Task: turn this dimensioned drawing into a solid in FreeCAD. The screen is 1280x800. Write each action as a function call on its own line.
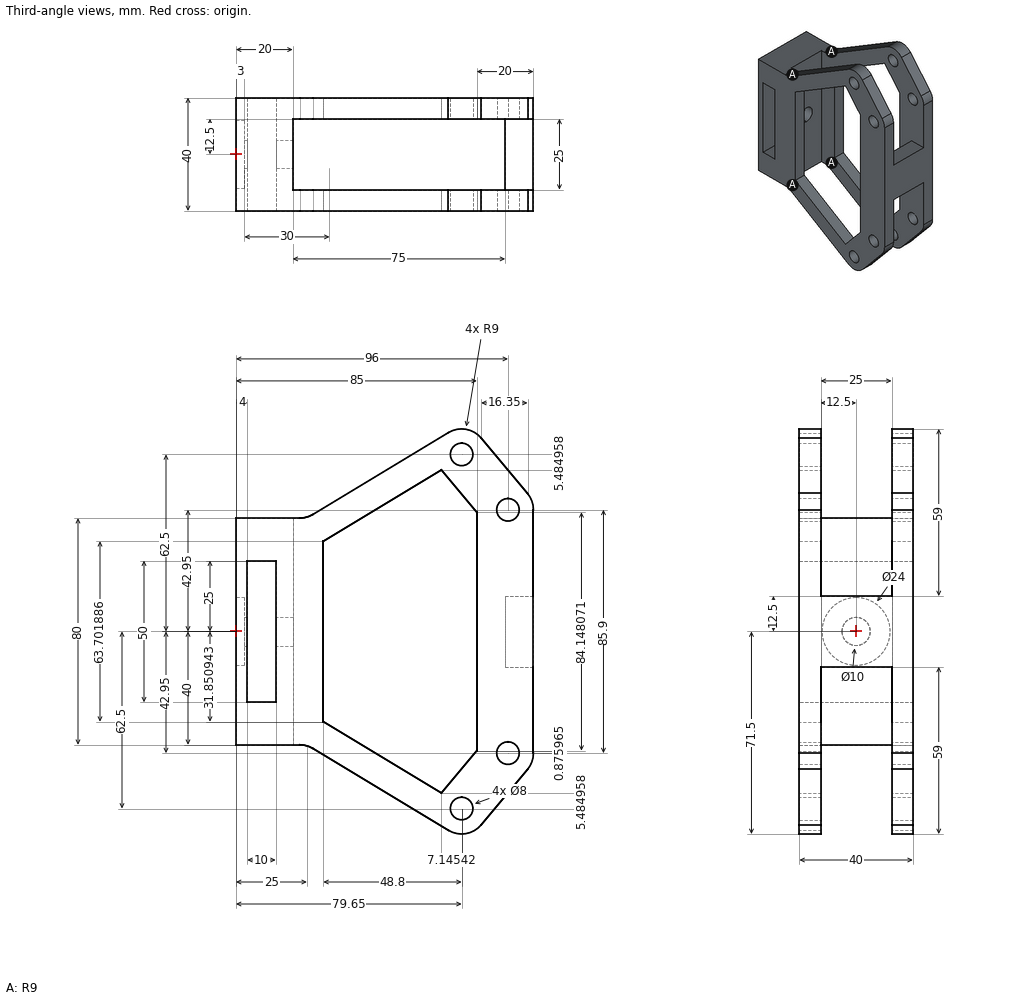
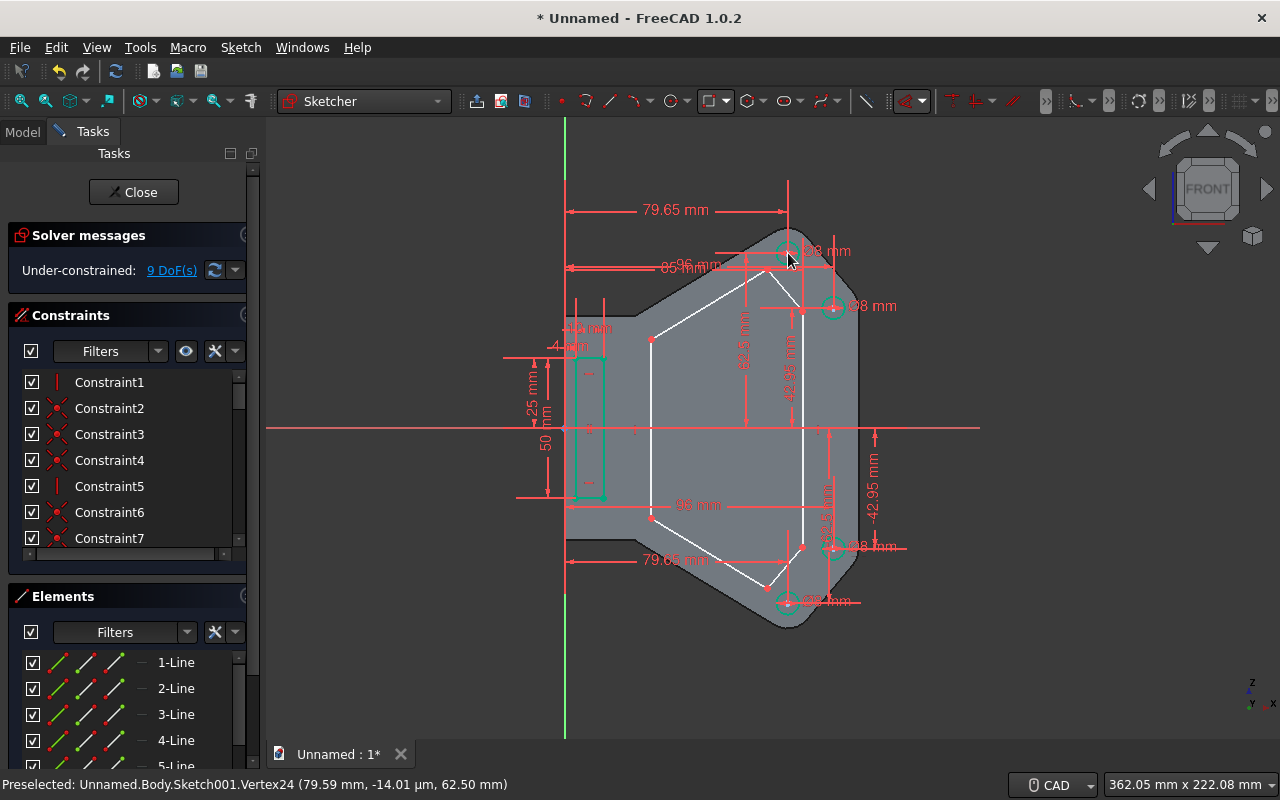
click(651, 518)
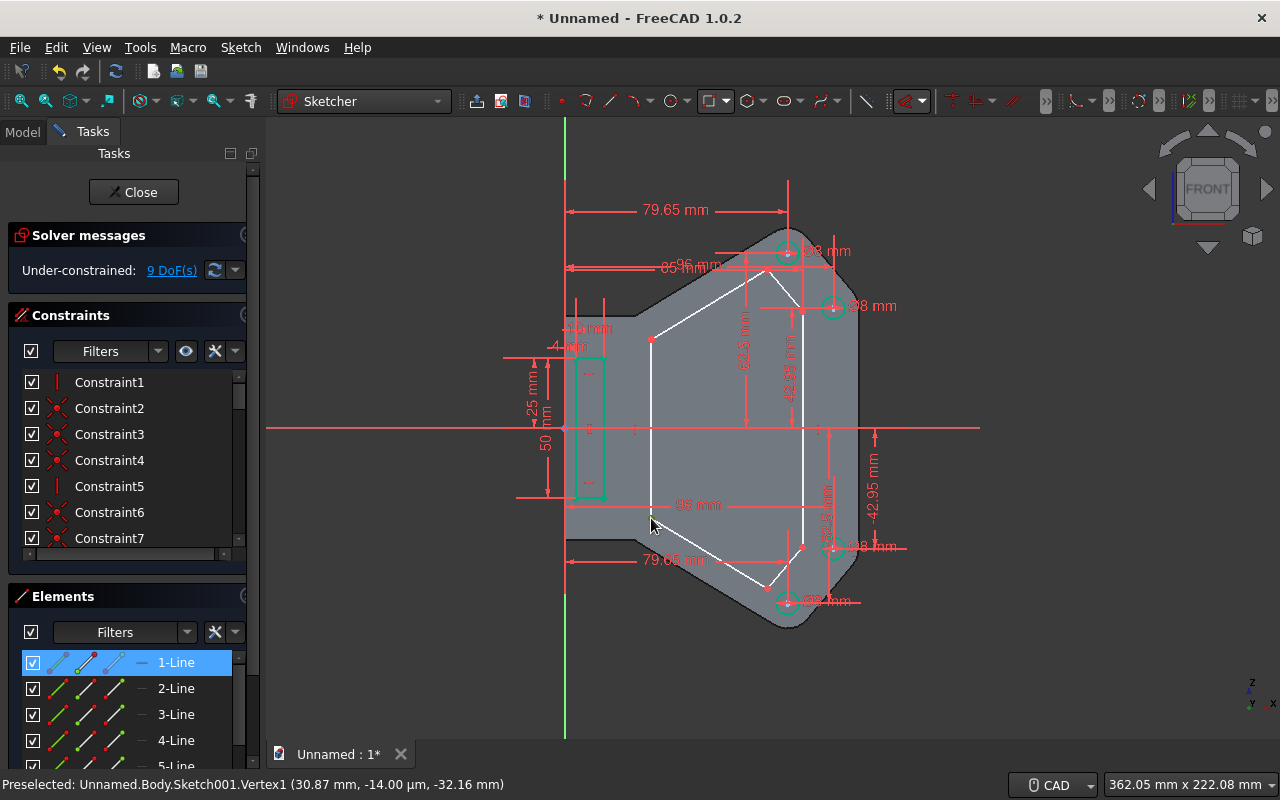
click(788, 603)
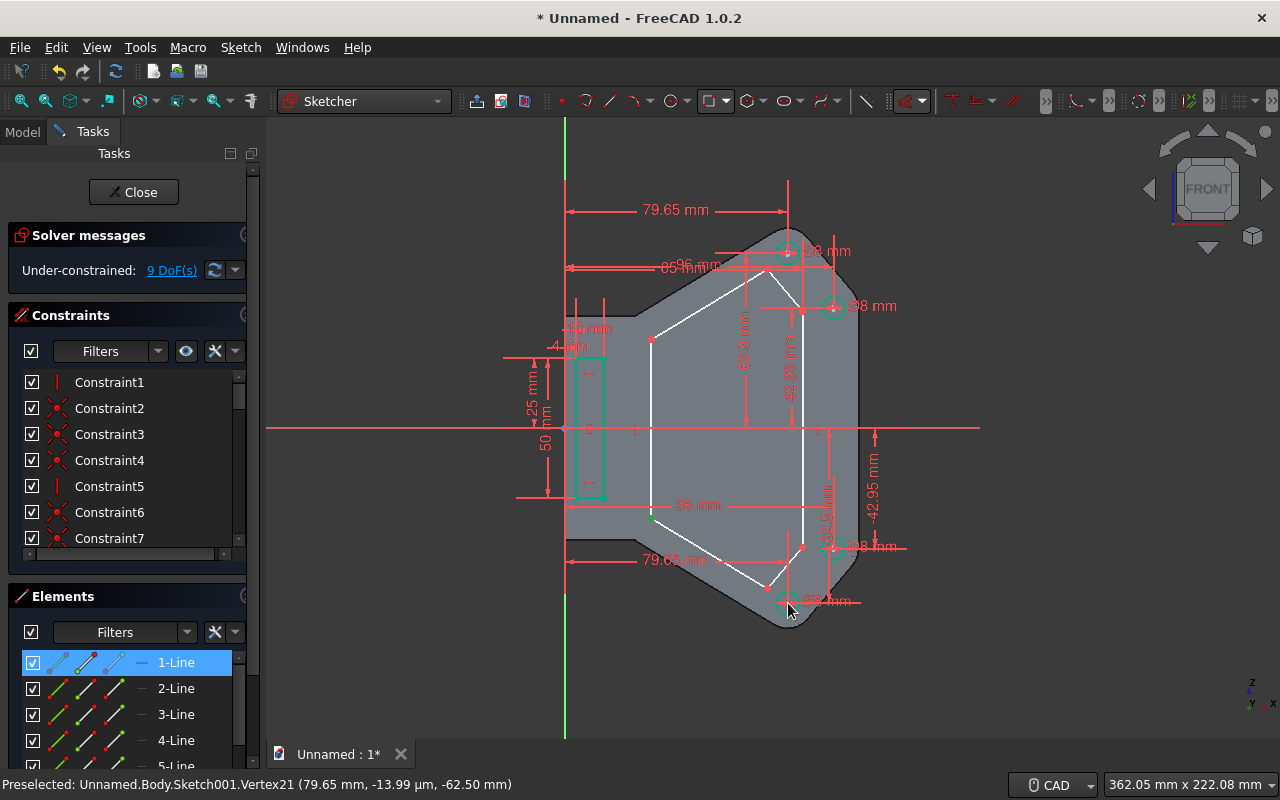
click(924, 102)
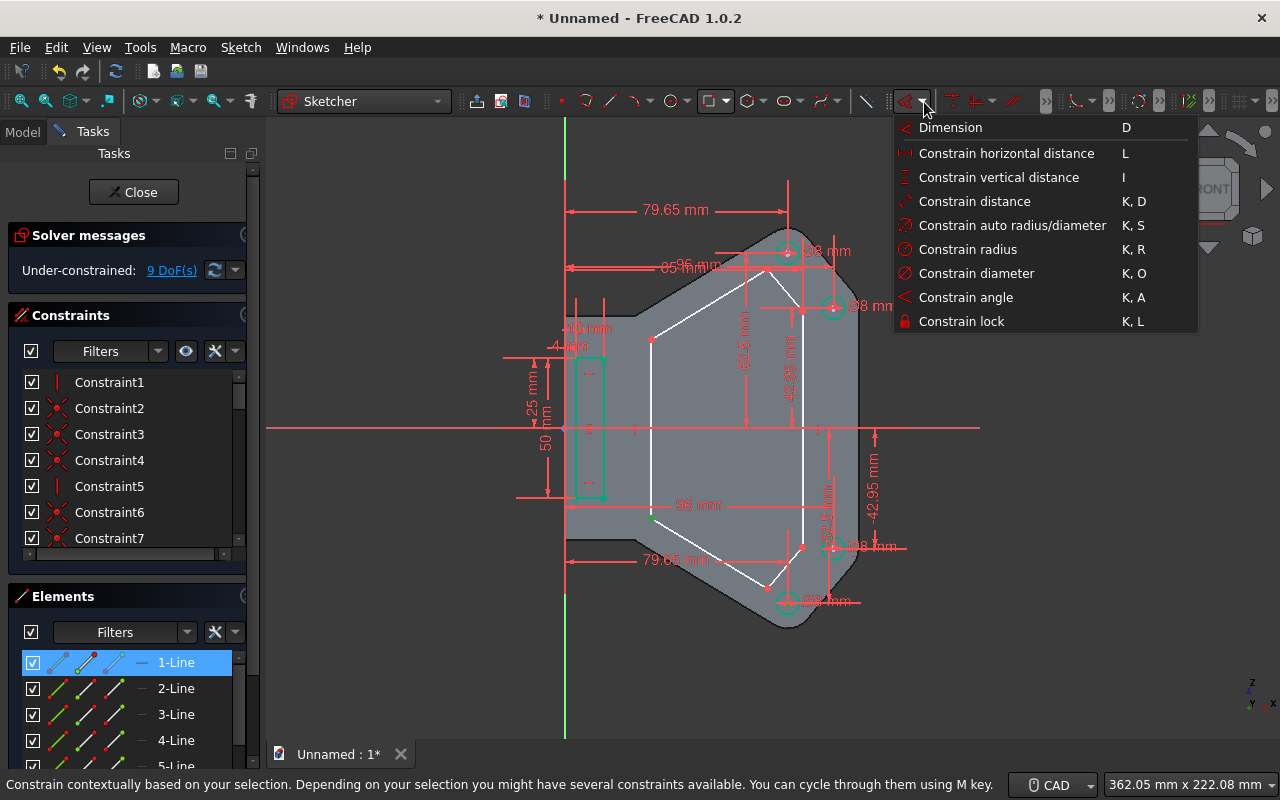
click(1046, 153)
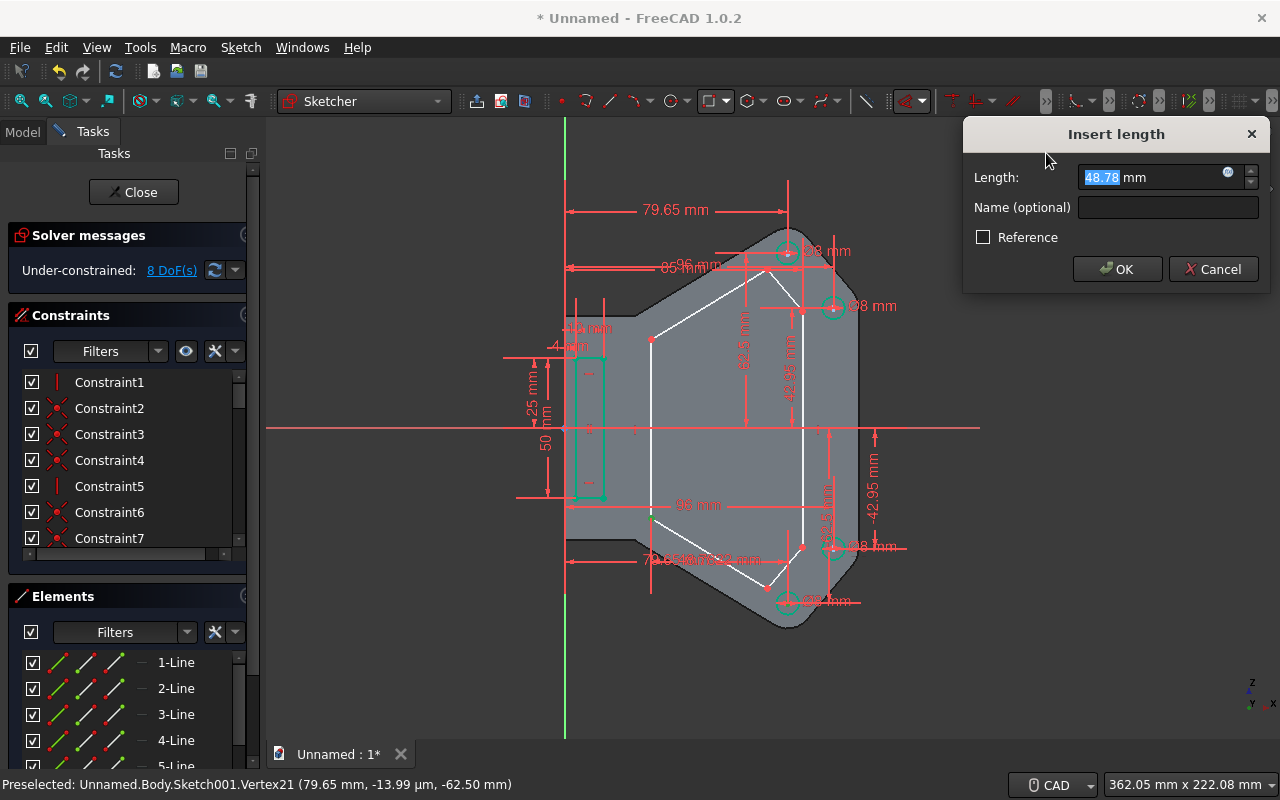
text(48.8)
key(Return)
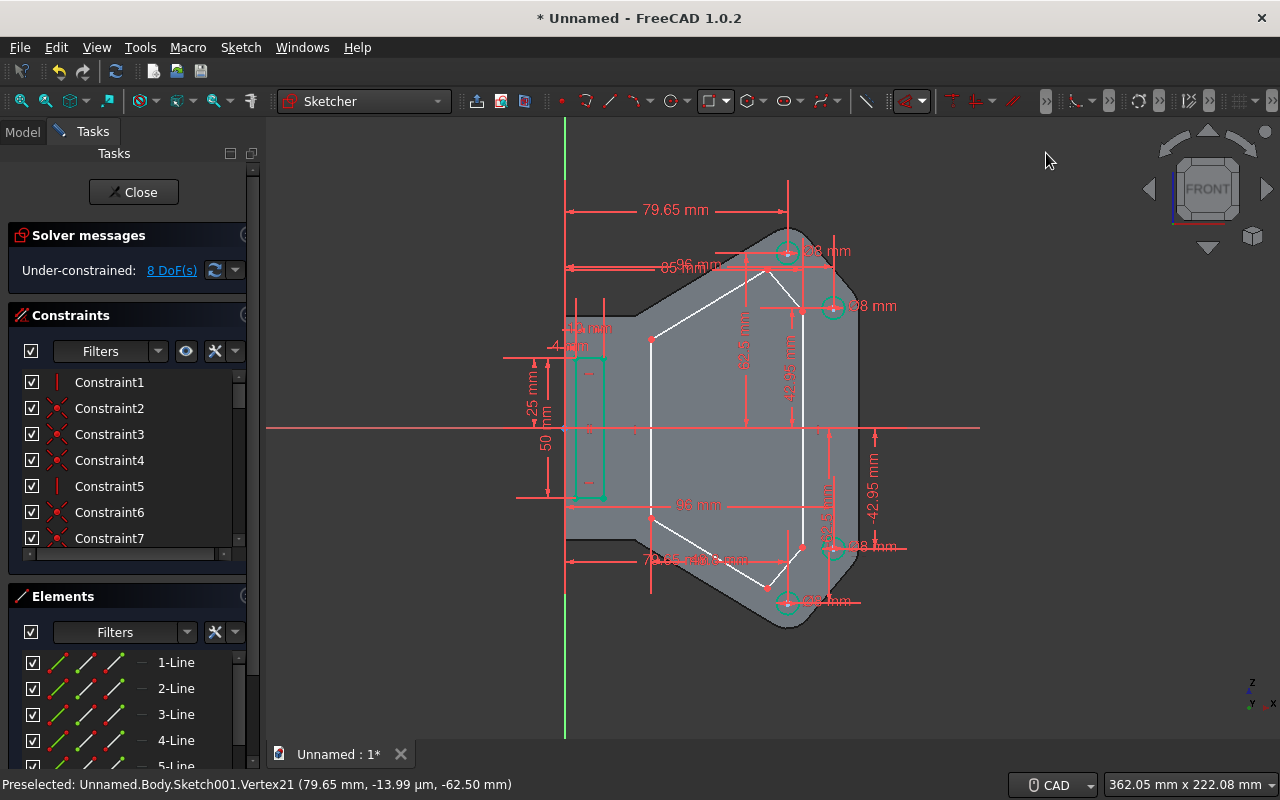
scroll(767, 589, up, 4)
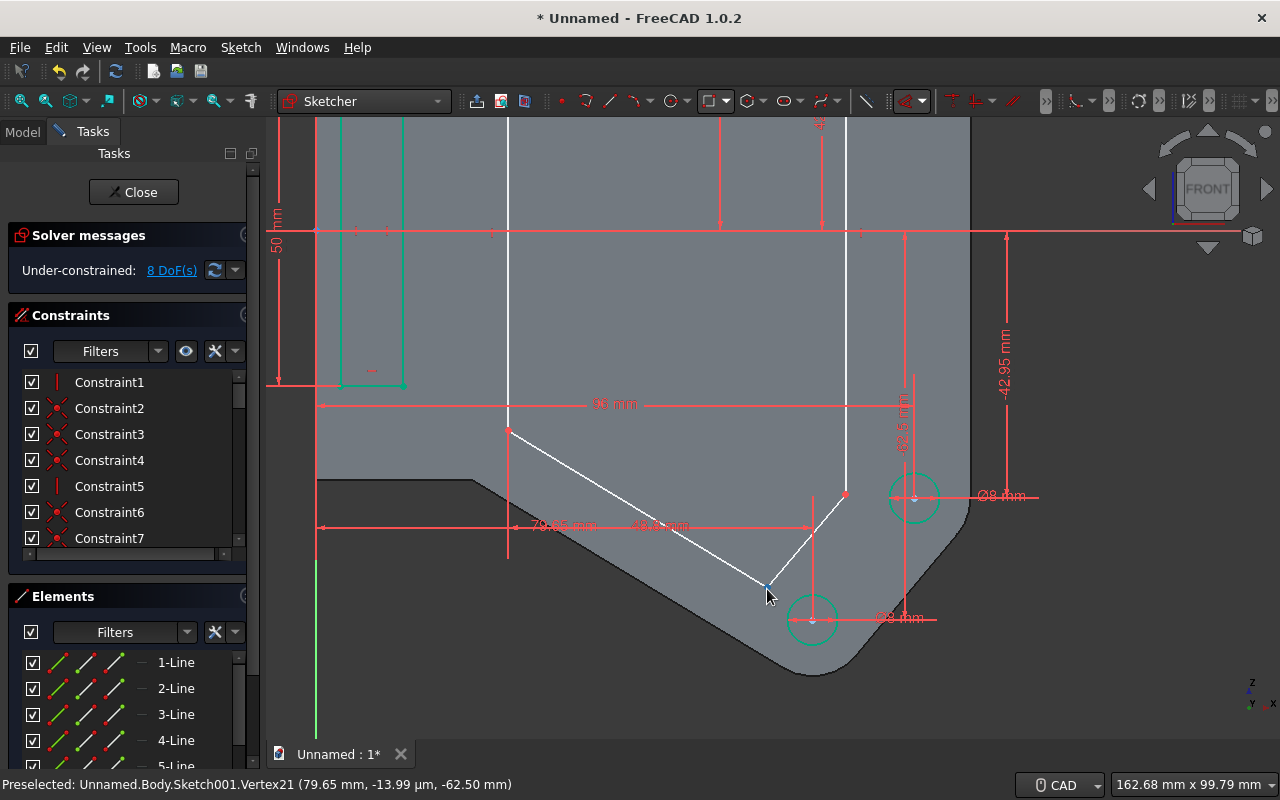
click(767, 588)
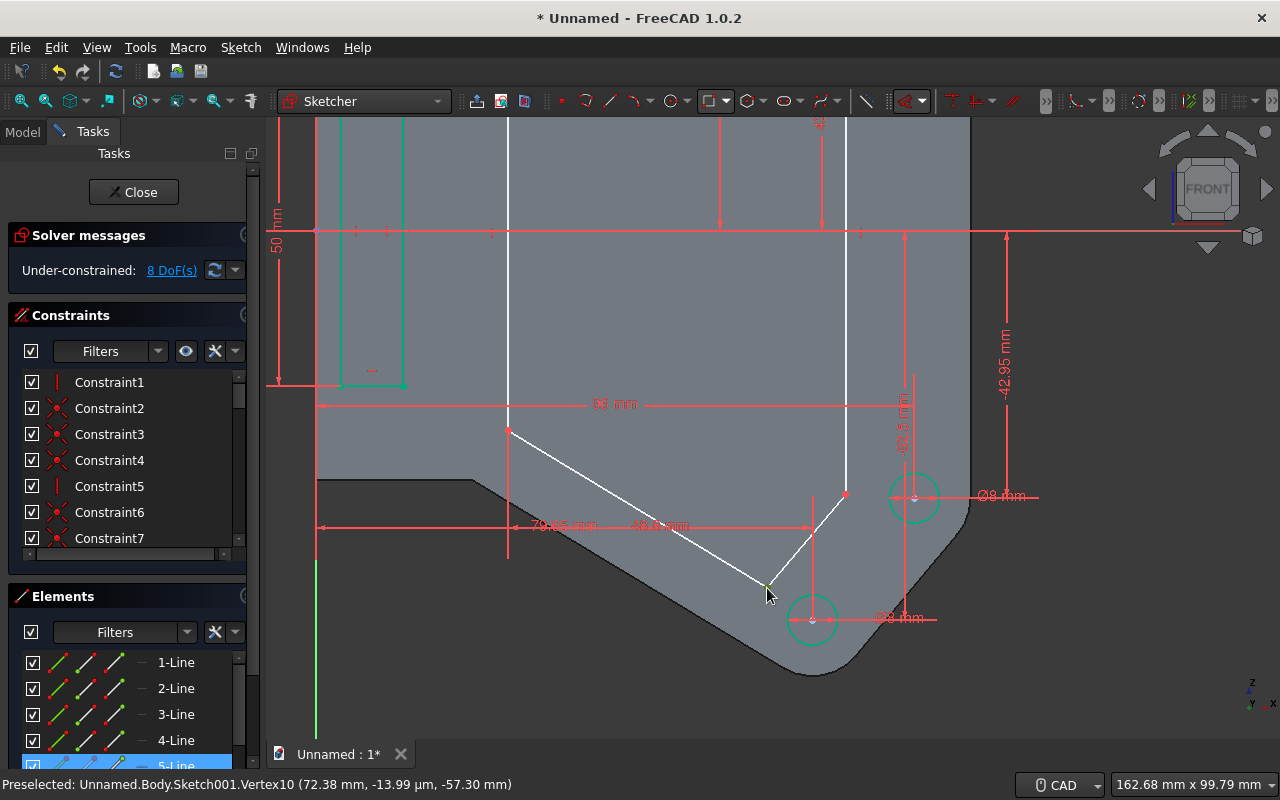
click(813, 620)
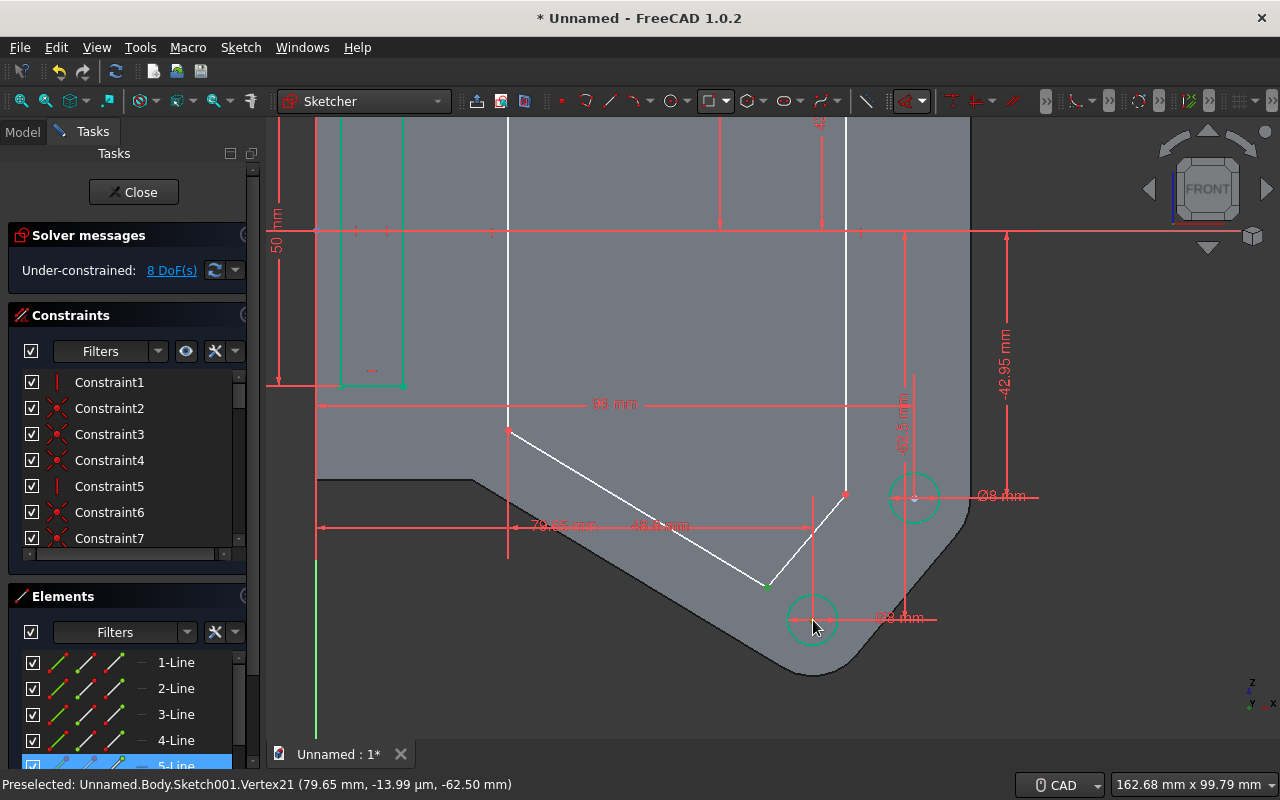
key(l)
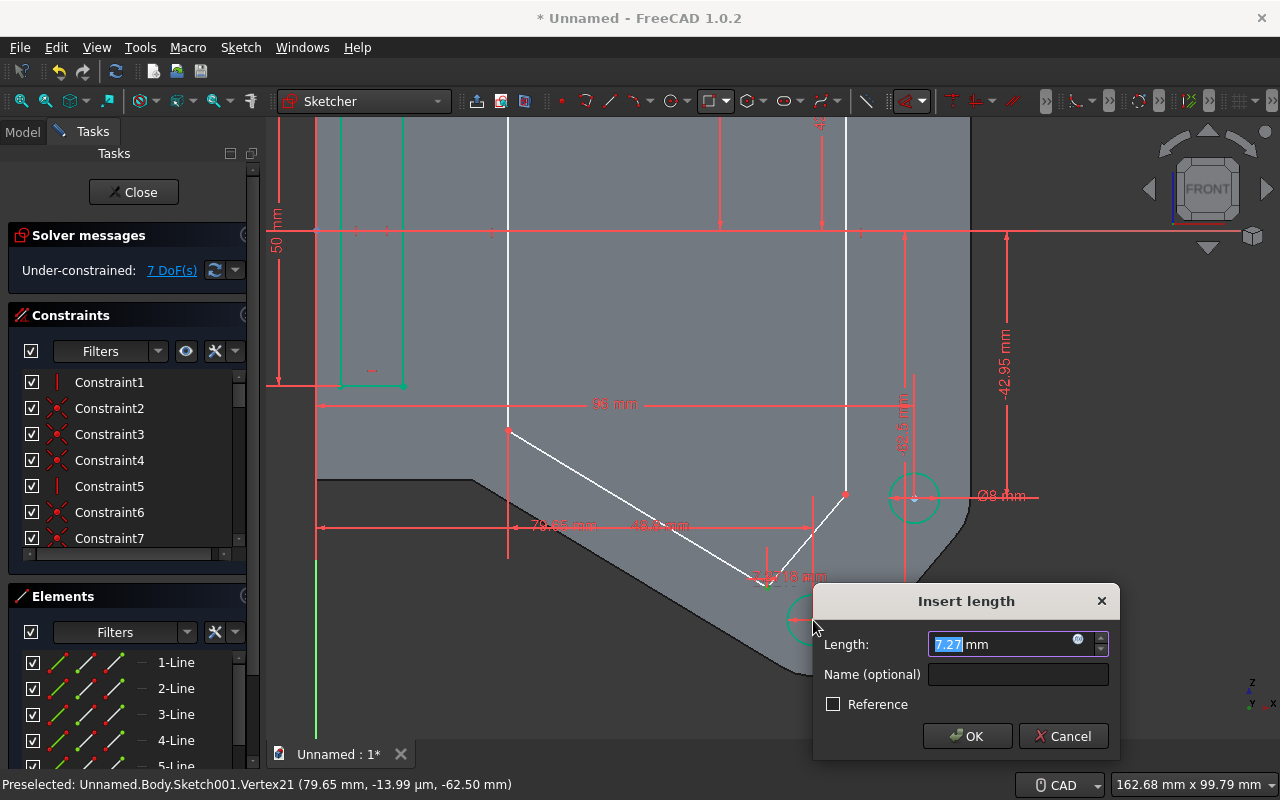
text(7.14542)
key(Return)